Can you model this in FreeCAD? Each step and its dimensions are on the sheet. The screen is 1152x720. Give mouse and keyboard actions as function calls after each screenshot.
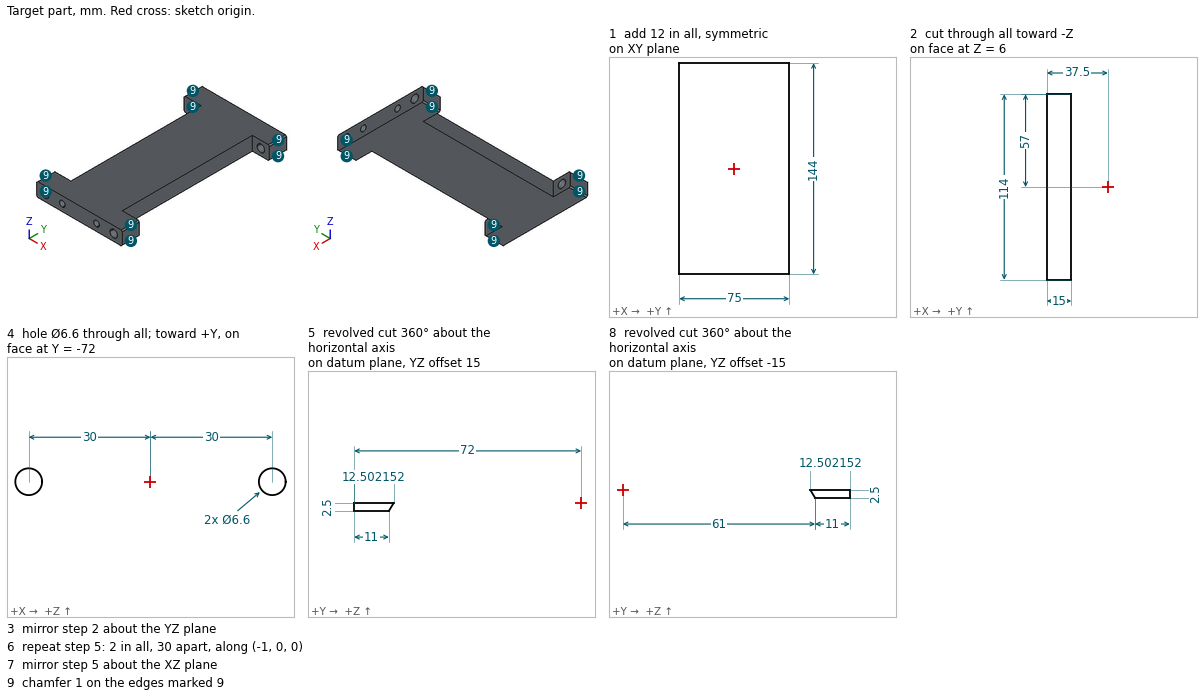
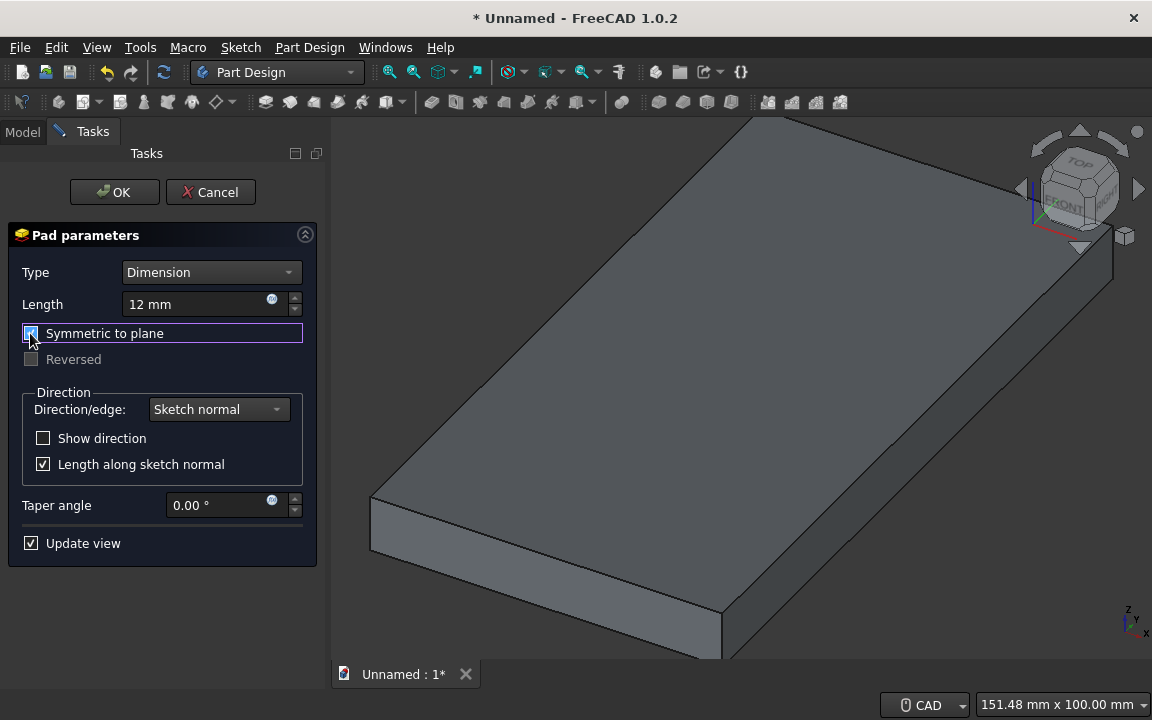
click(115, 192)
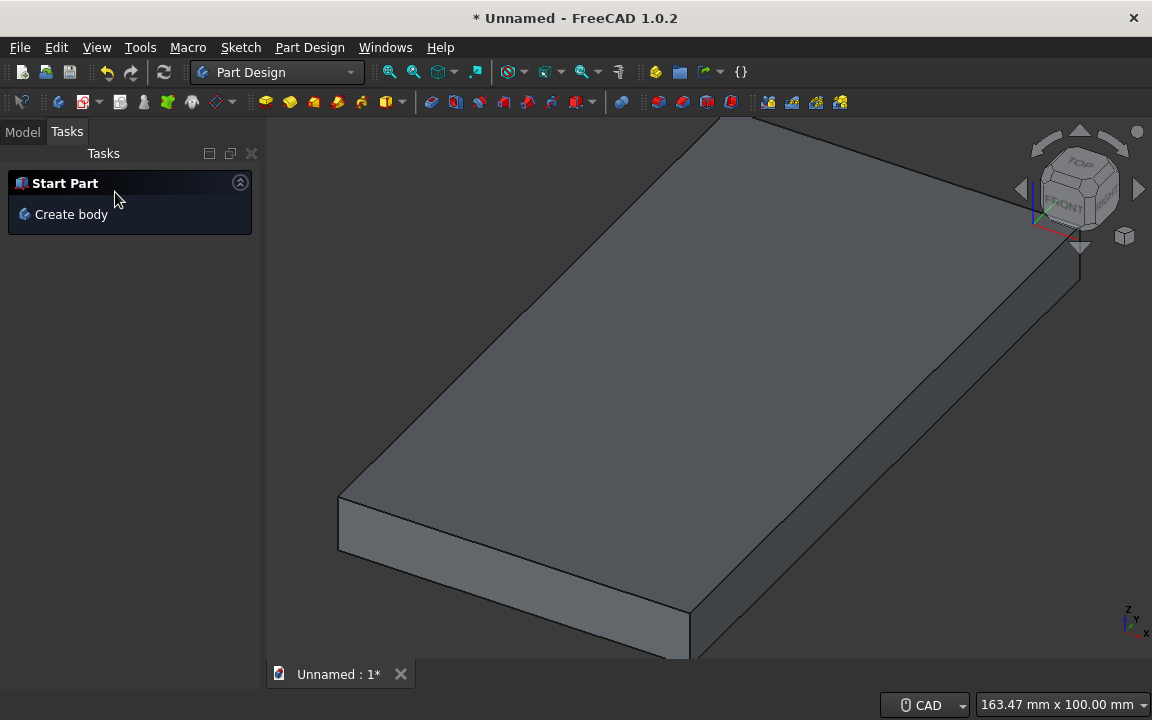
click(390, 72)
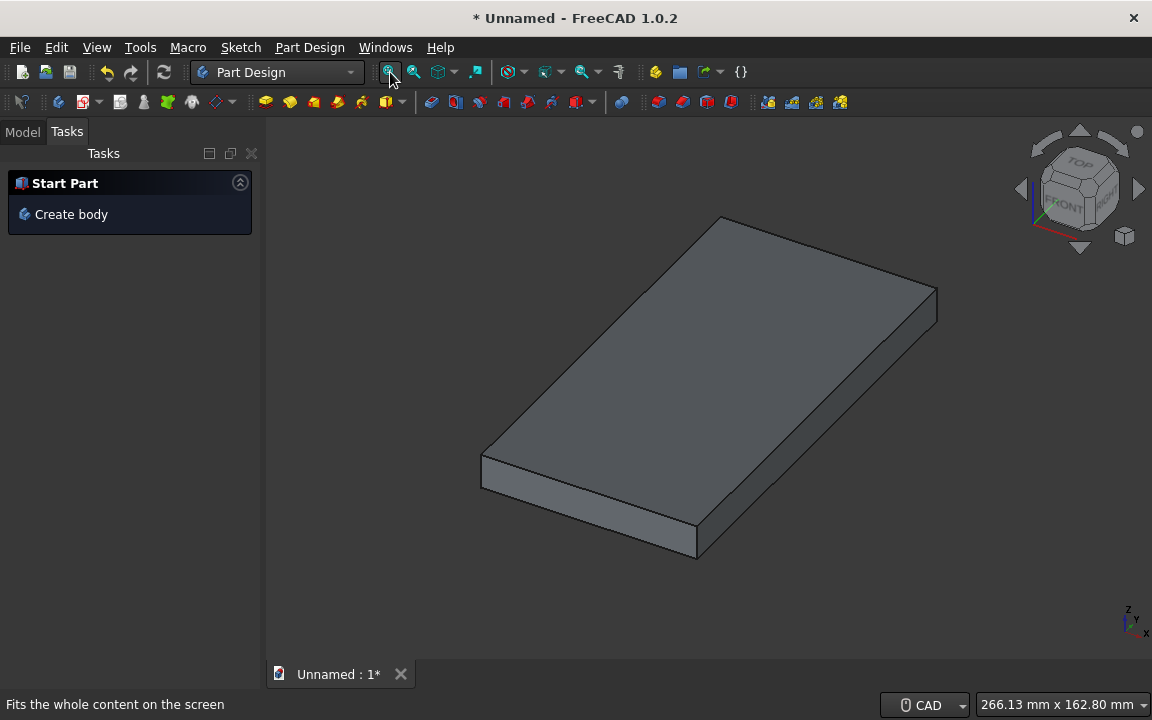
click(743, 337)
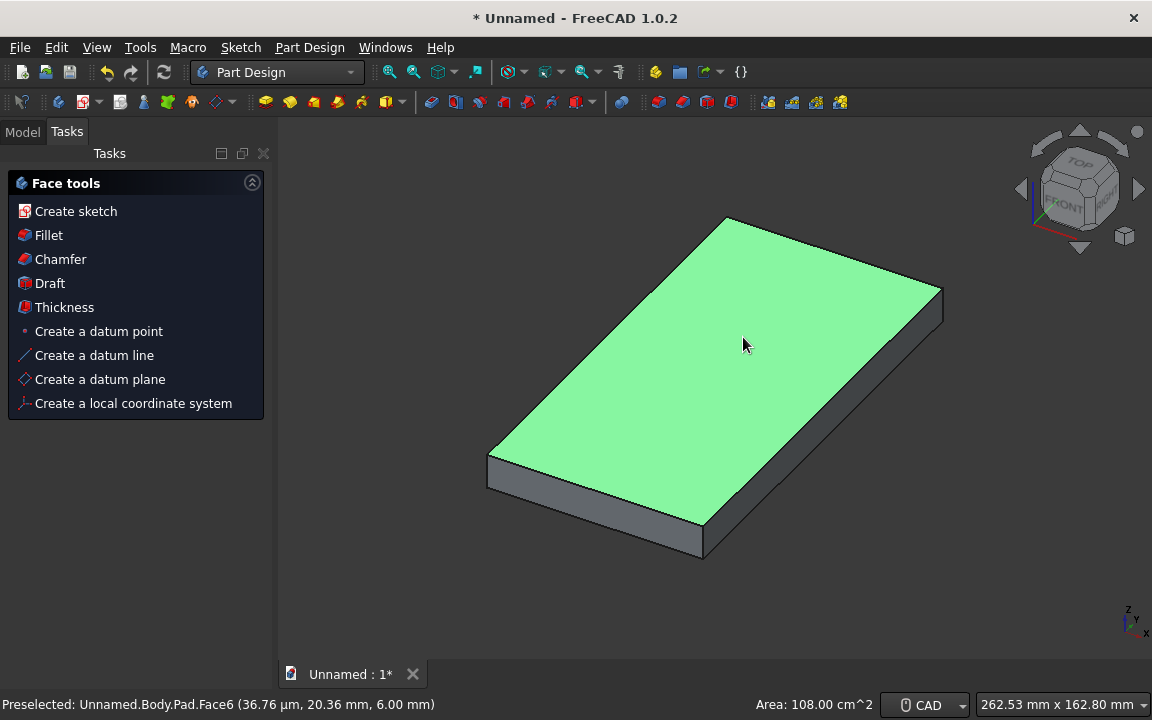
click(84, 102)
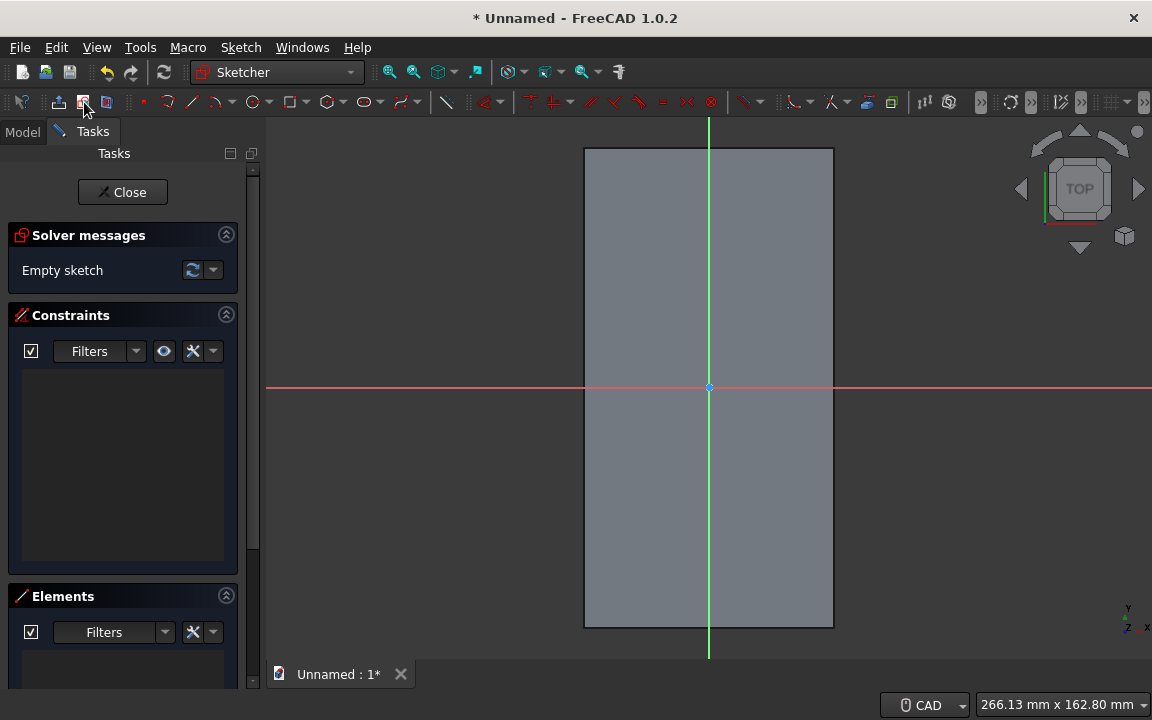
key(g)
key(r)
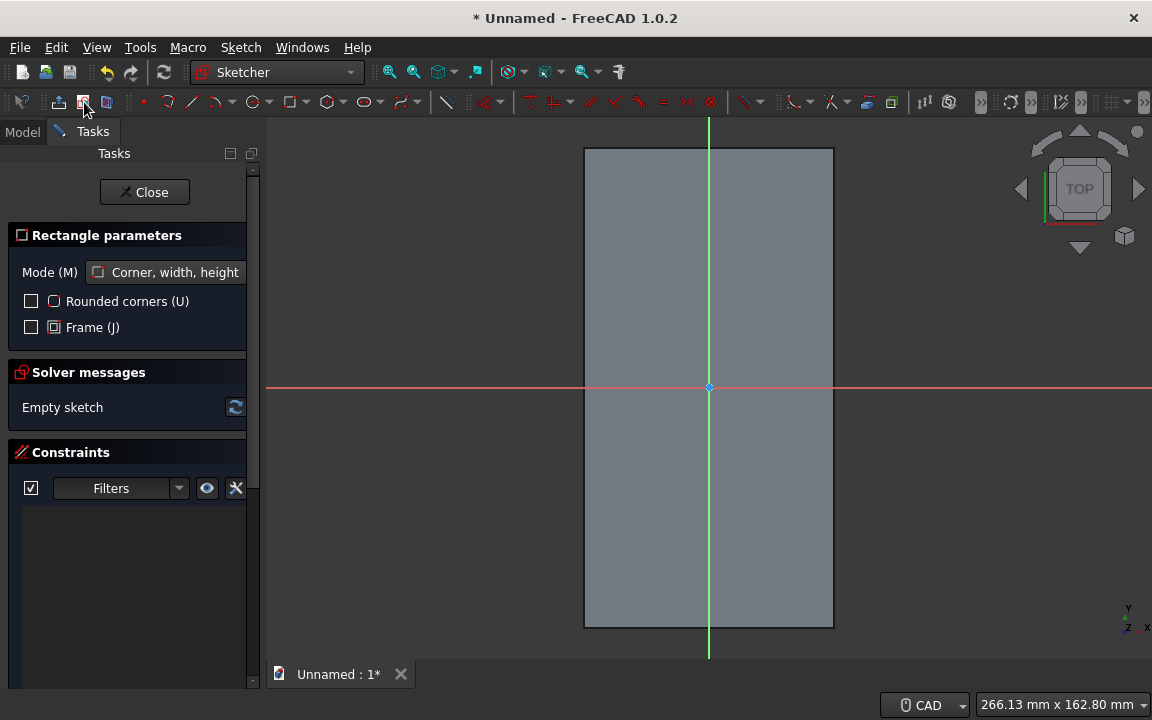
click(584, 198)
move(634, 578)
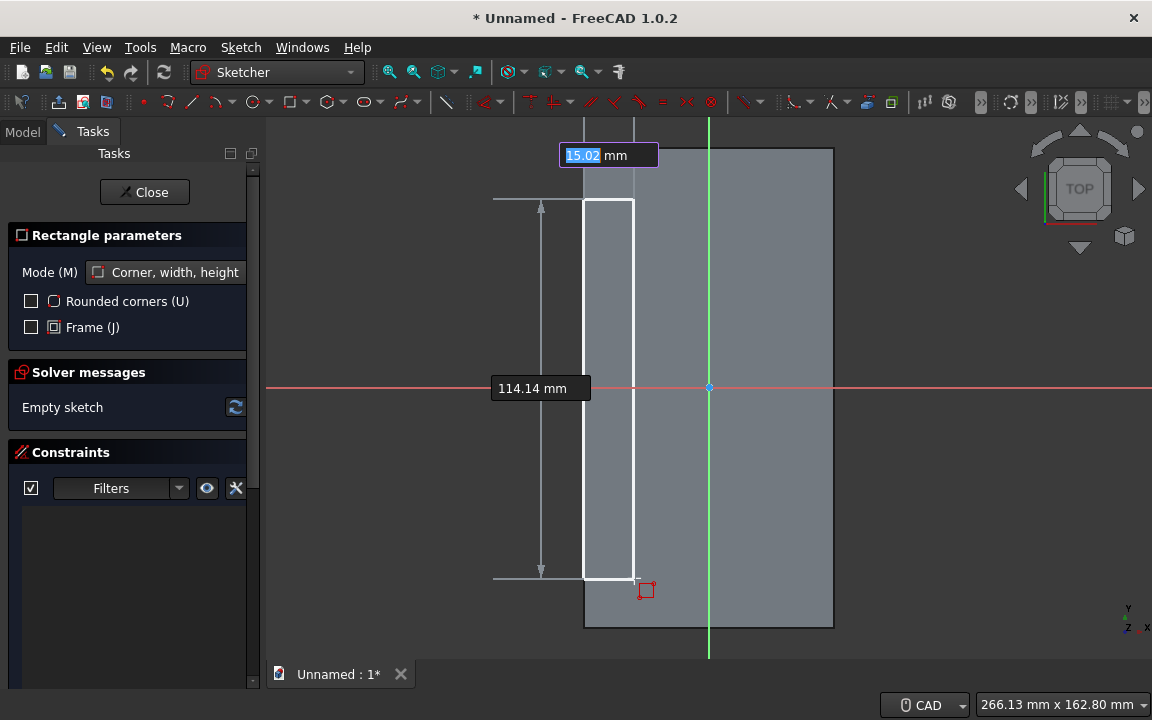
text(15)
key(Tab)
text(114)
key(Return)
key(Escape)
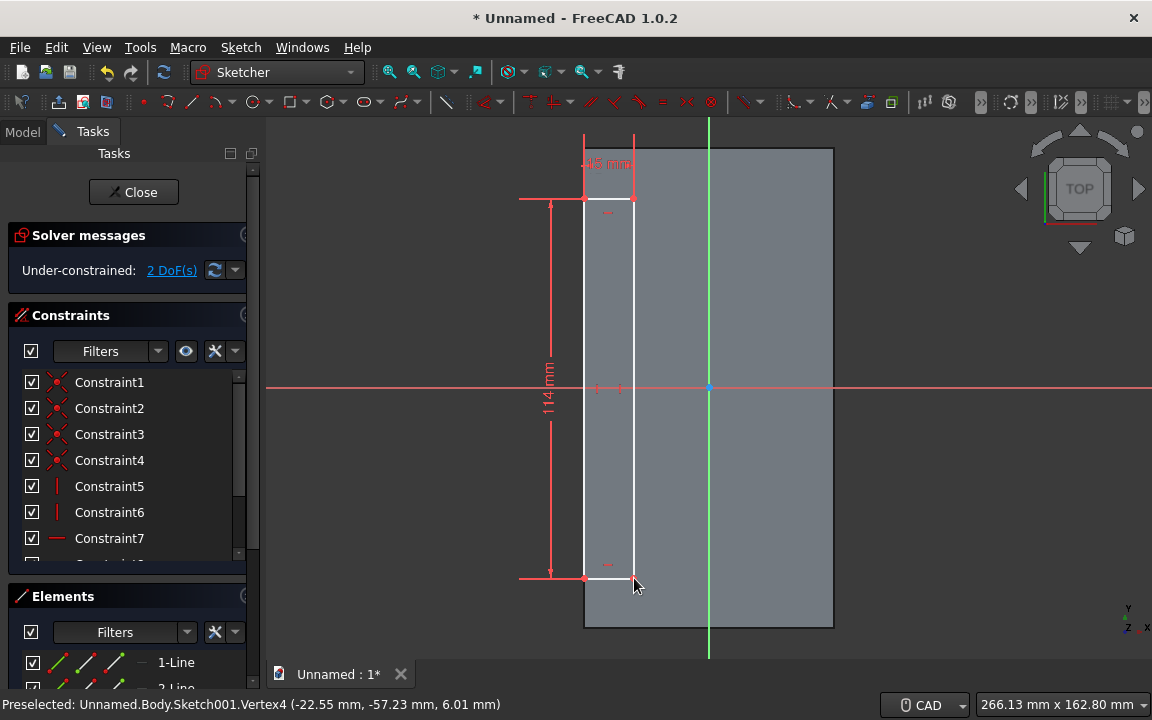
click(484, 102)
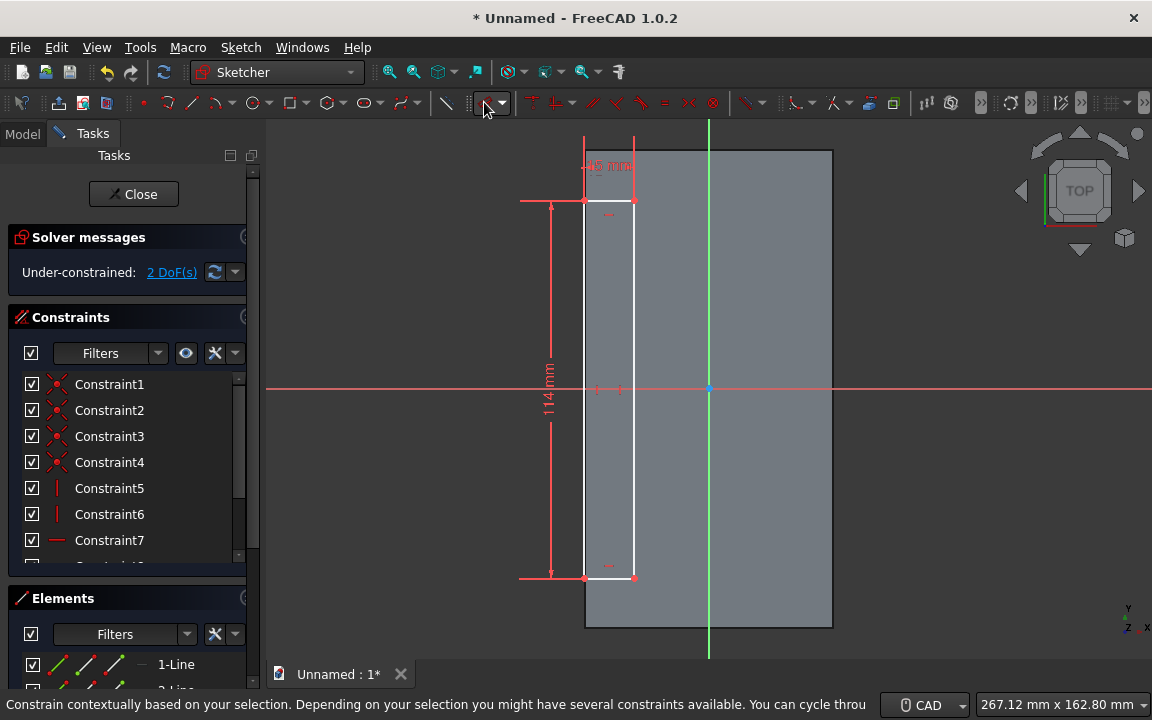
click(584, 201)
click(550, 295)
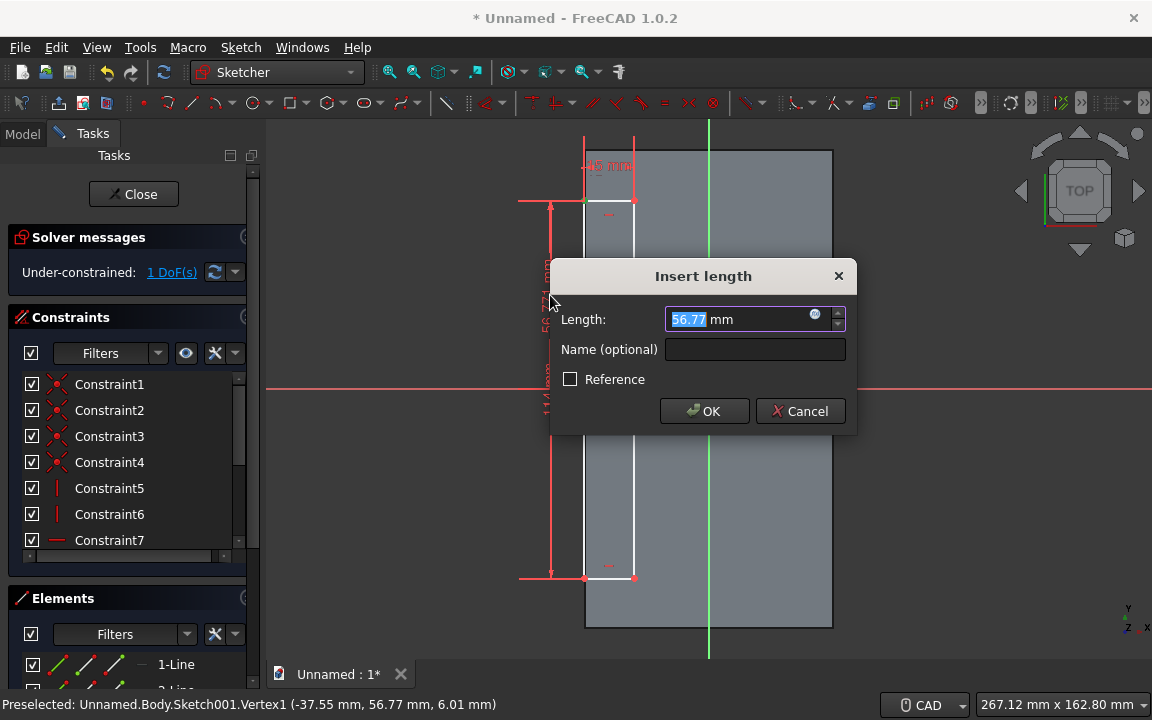
text(57)
key(Return)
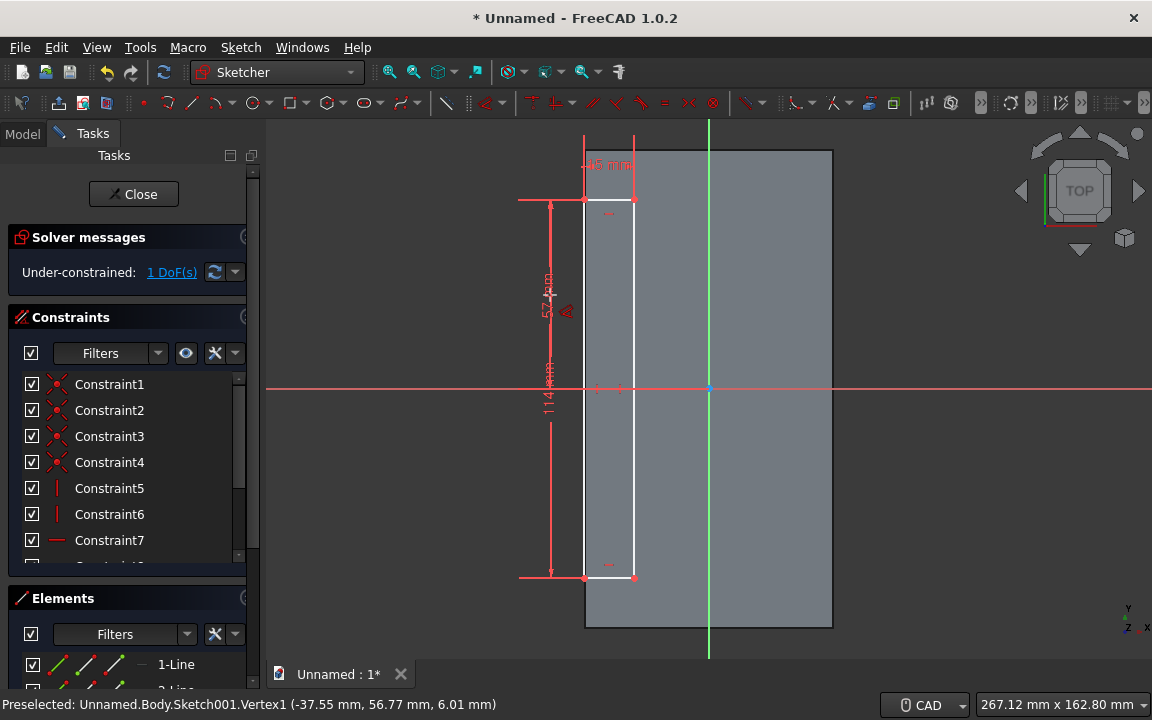
click(584, 200)
click(647, 166)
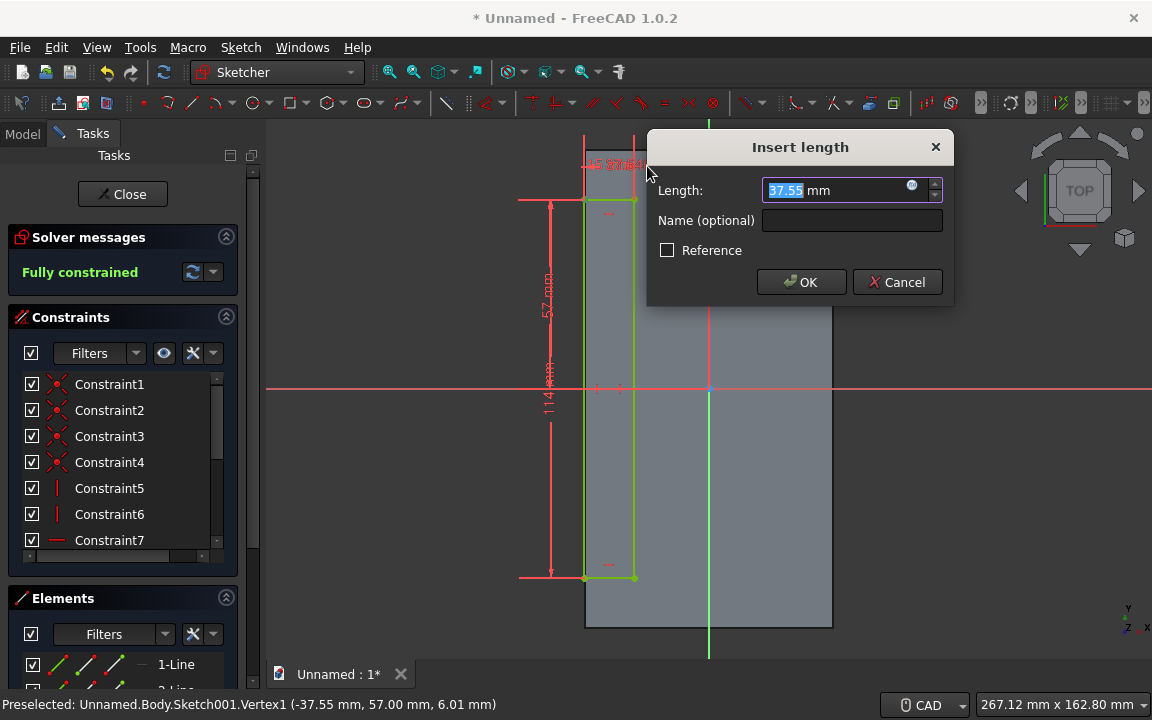
text(37.5)
key(Return)
key(Escape)